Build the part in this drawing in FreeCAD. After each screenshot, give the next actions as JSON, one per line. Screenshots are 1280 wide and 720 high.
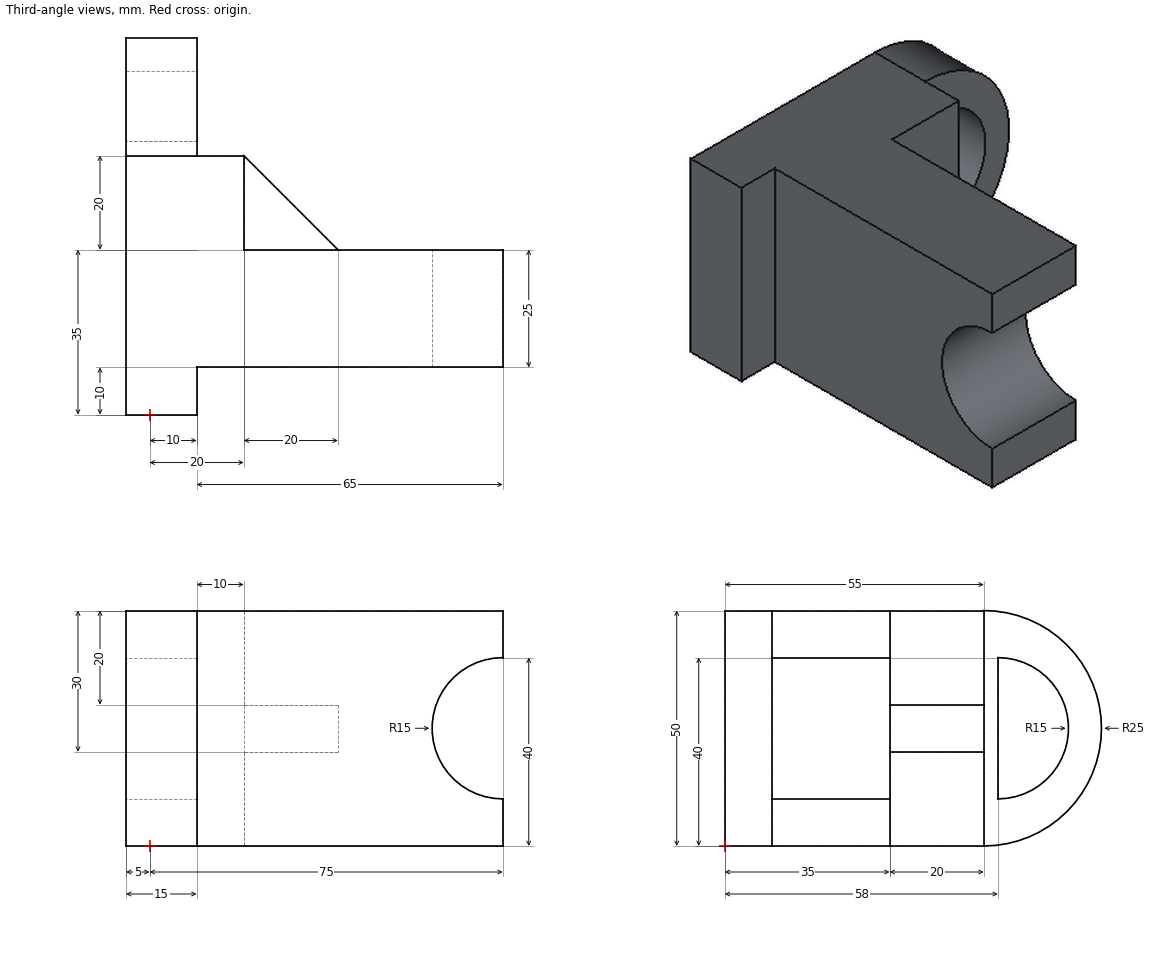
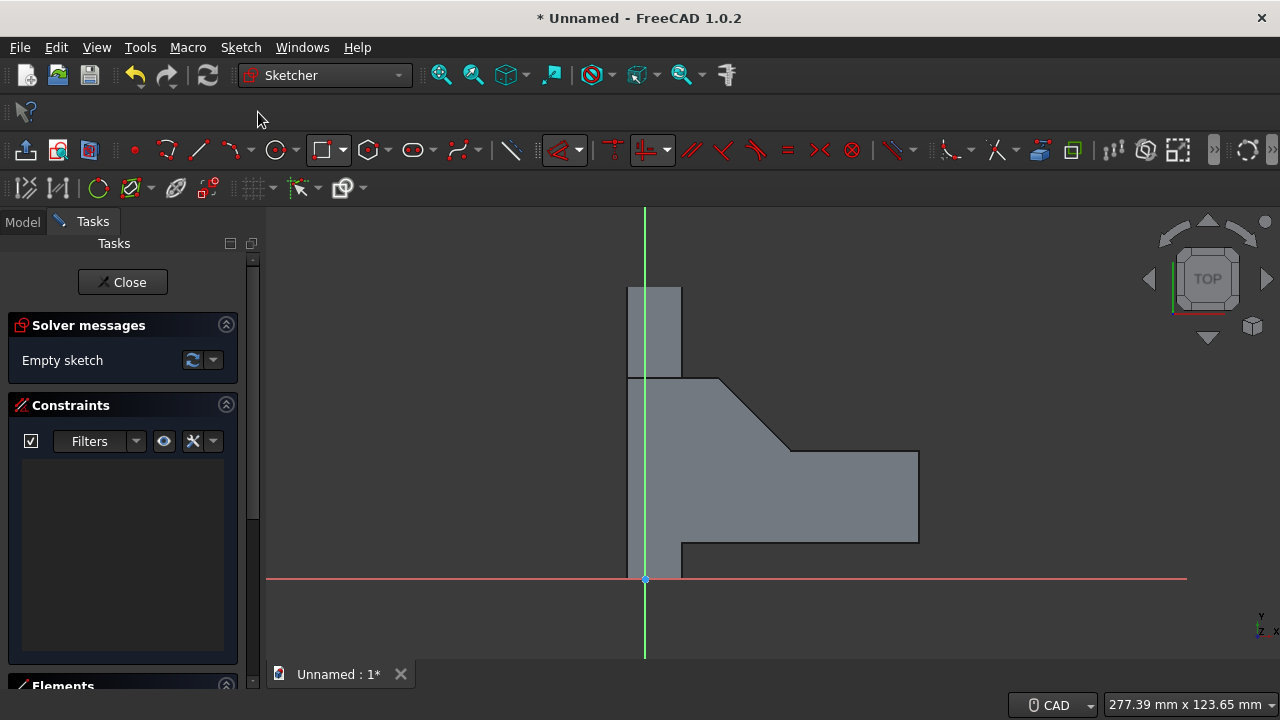
{"action": "scroll", "coordinate": [771, 409], "scroll_direction": "up", "scroll_amount": 7}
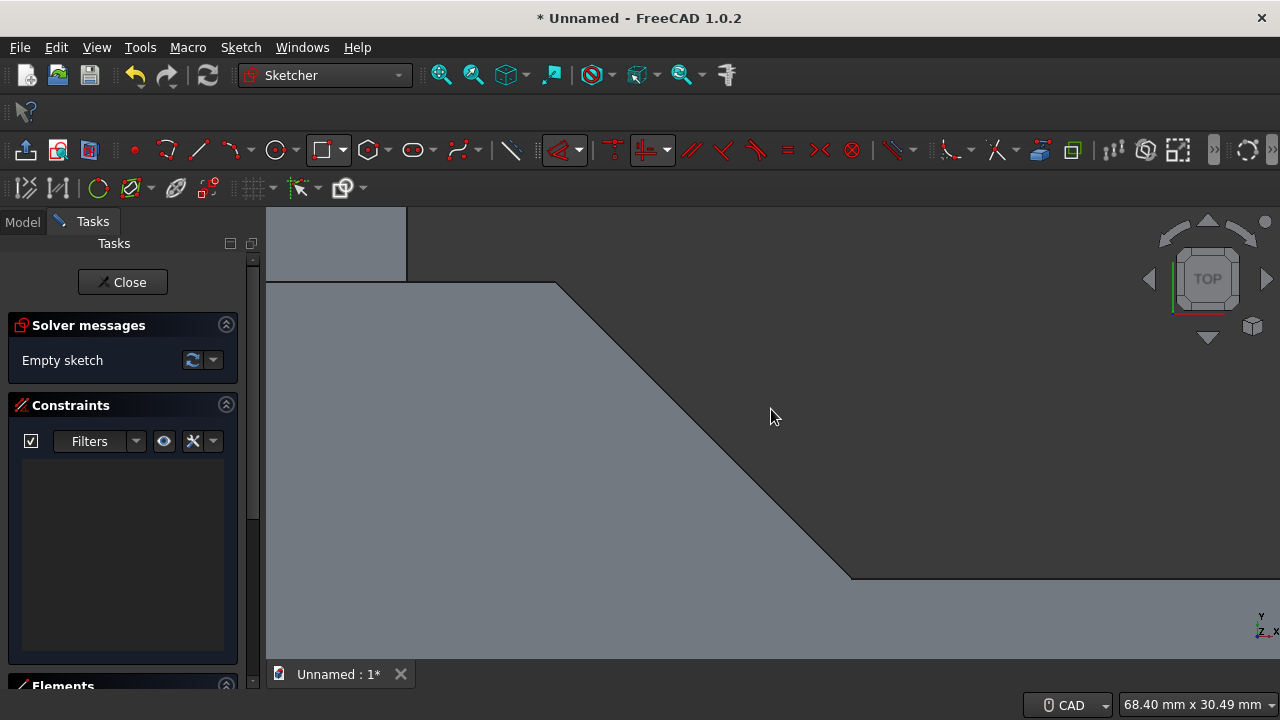
{"action": "left_click", "coordinate": [168, 150]}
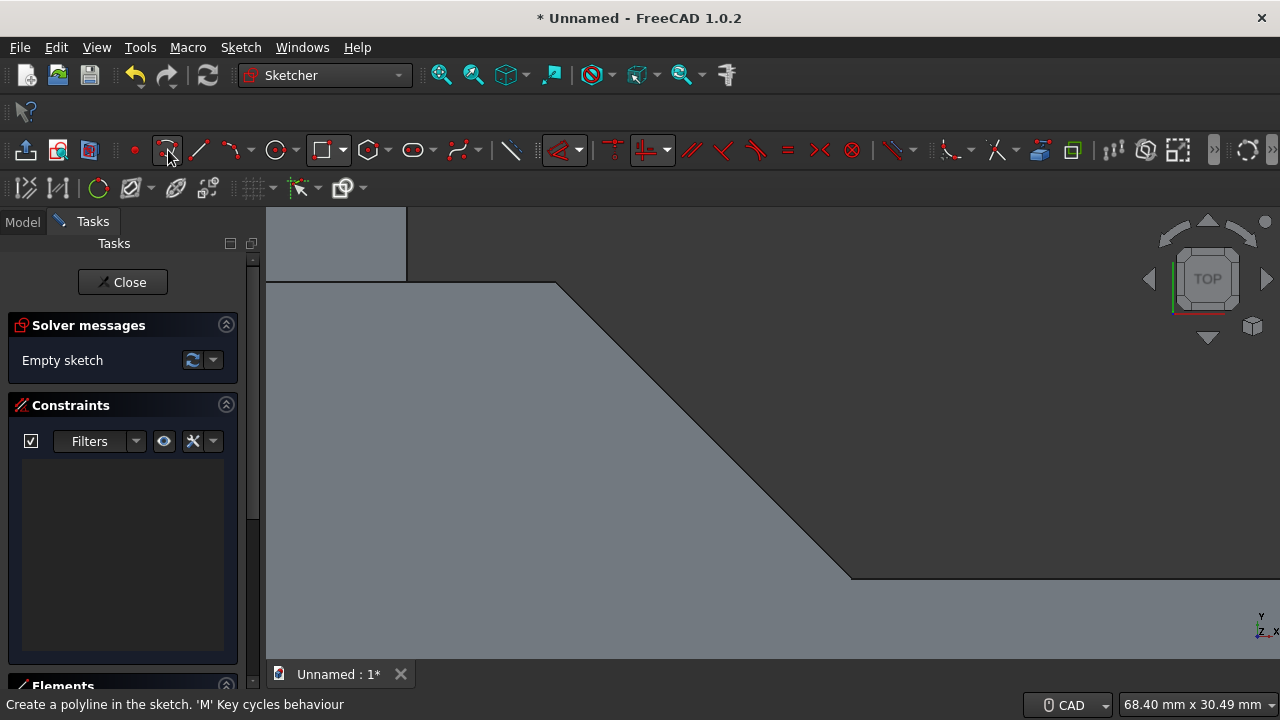
{"action": "left_click", "coordinate": [555, 579]}
{"action": "left_click", "coordinate": [852, 579]}
{"action": "left_click", "coordinate": [555, 282]}
{"action": "left_click", "coordinate": [555, 580]}
{"action": "key", "text": "Escape"}
{"action": "key", "text": "Escape"}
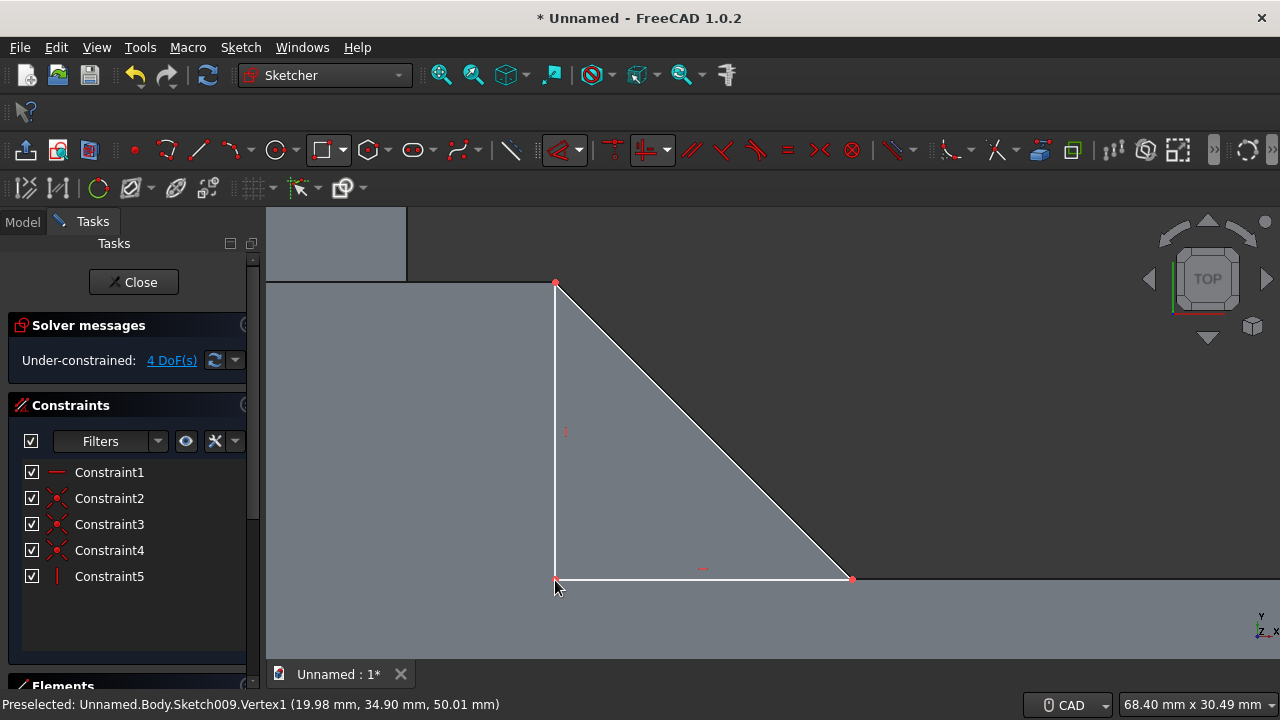
{"action": "left_click", "coordinate": [644, 580]}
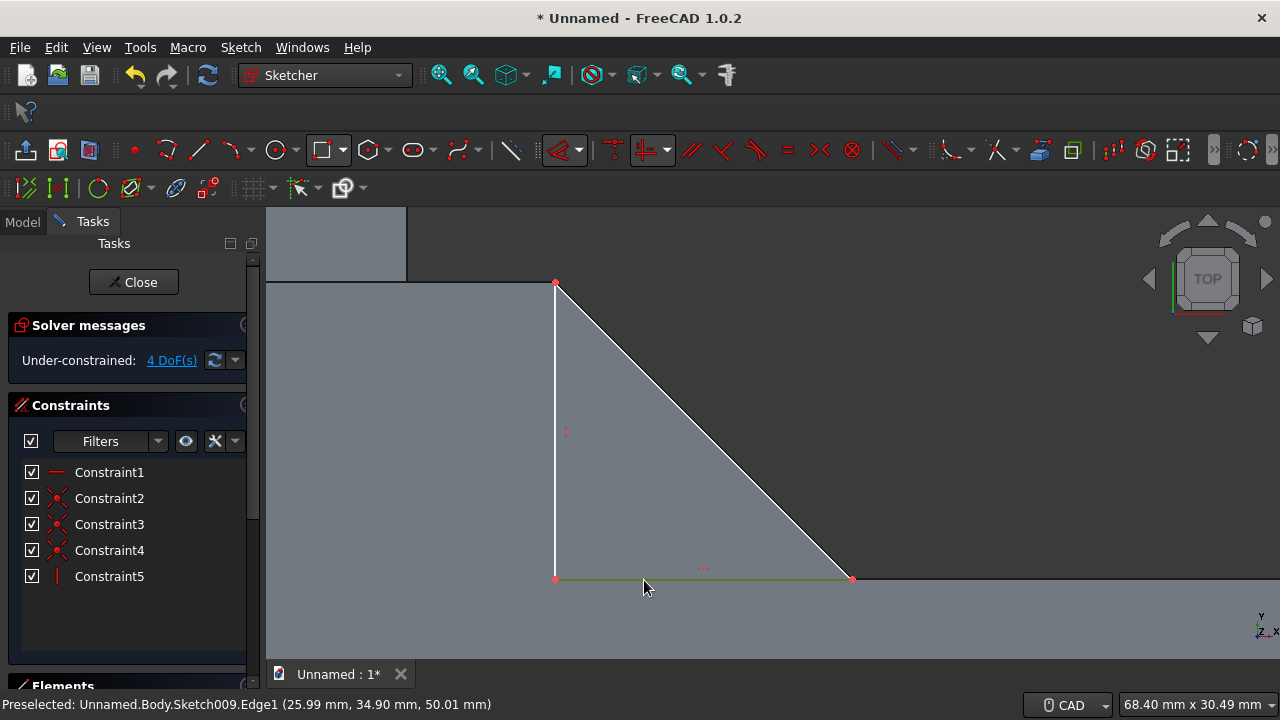
{"action": "left_click", "coordinate": [582, 150]}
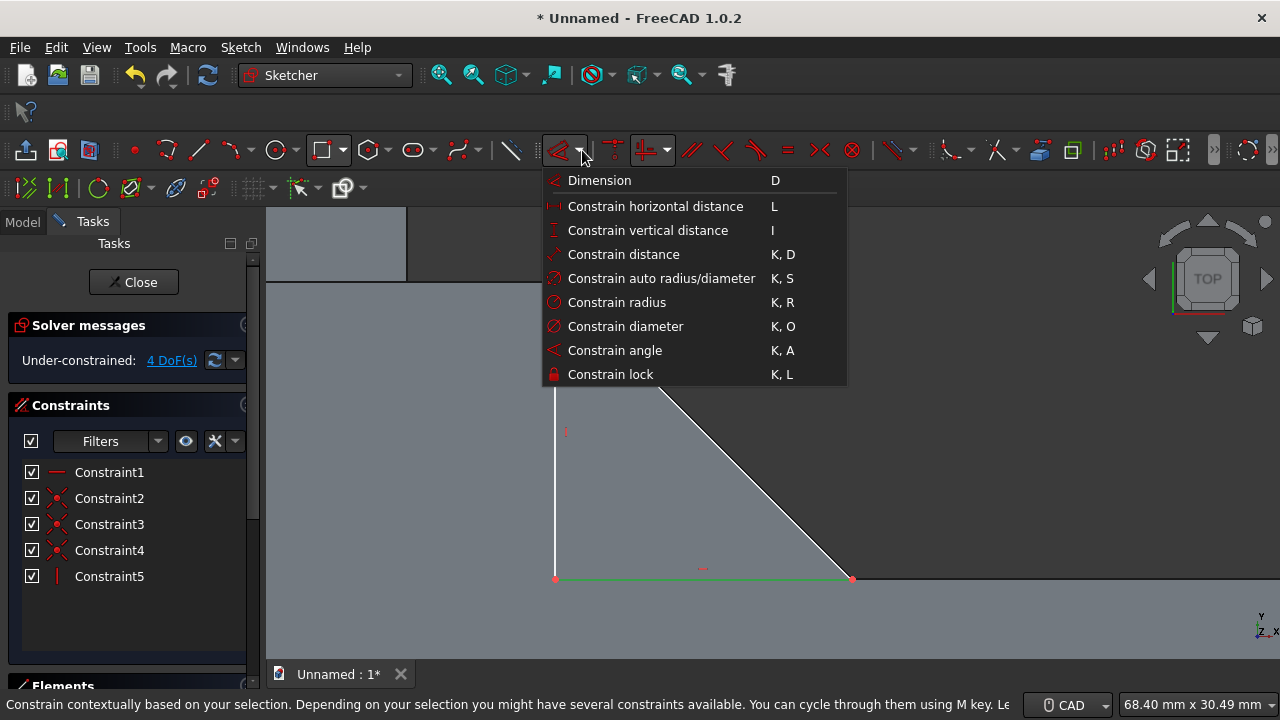
{"action": "left_click", "coordinate": [695, 206]}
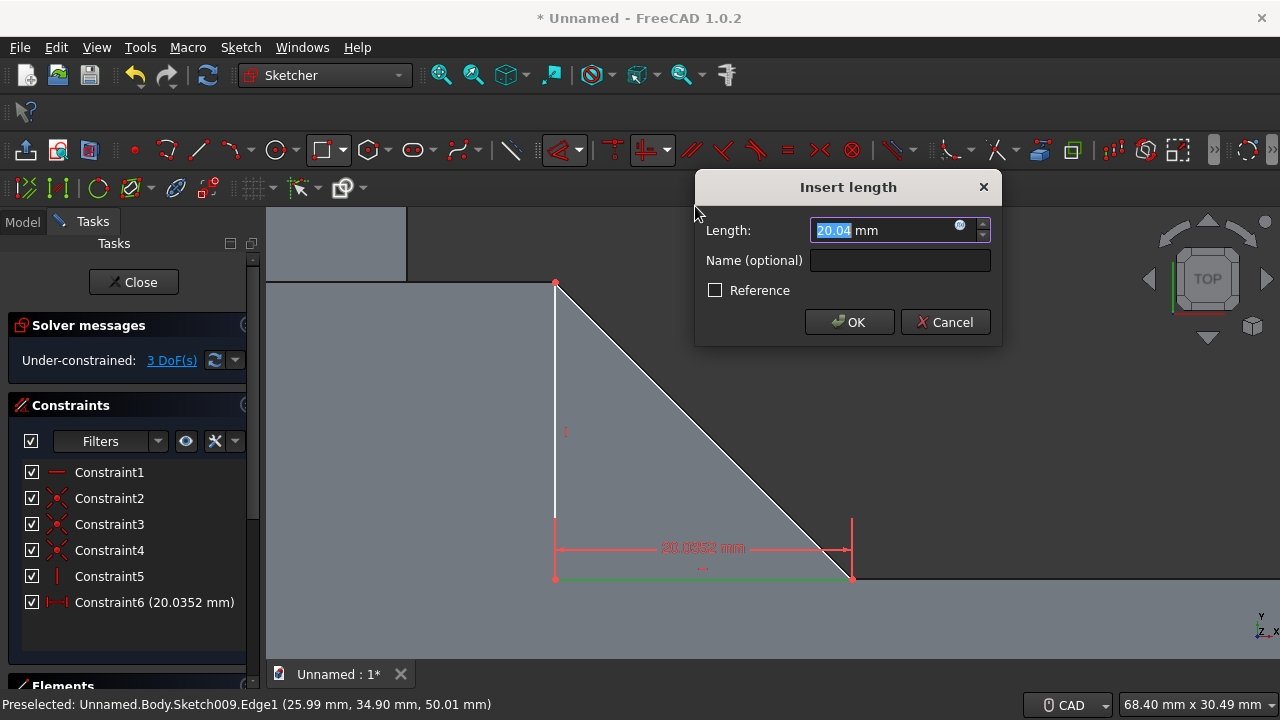
{"action": "type", "text": "20"}
{"action": "key", "text": "Return"}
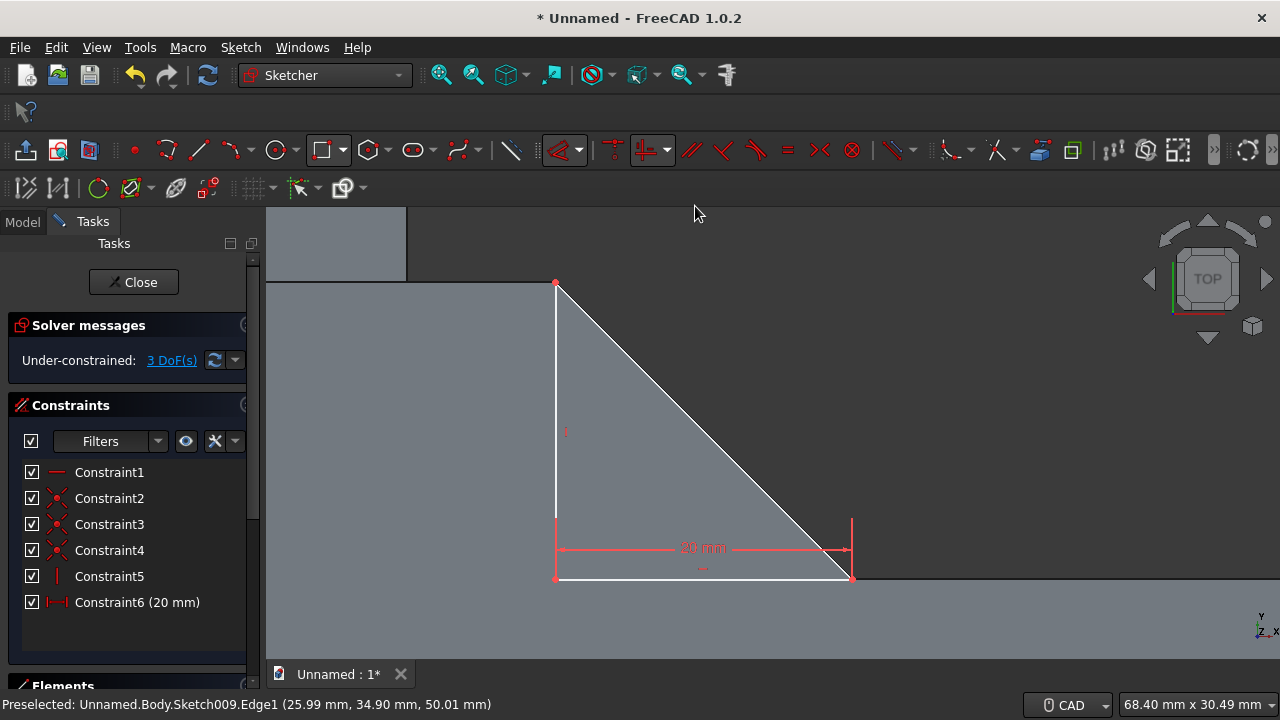
{"action": "left_click", "coordinate": [556, 372]}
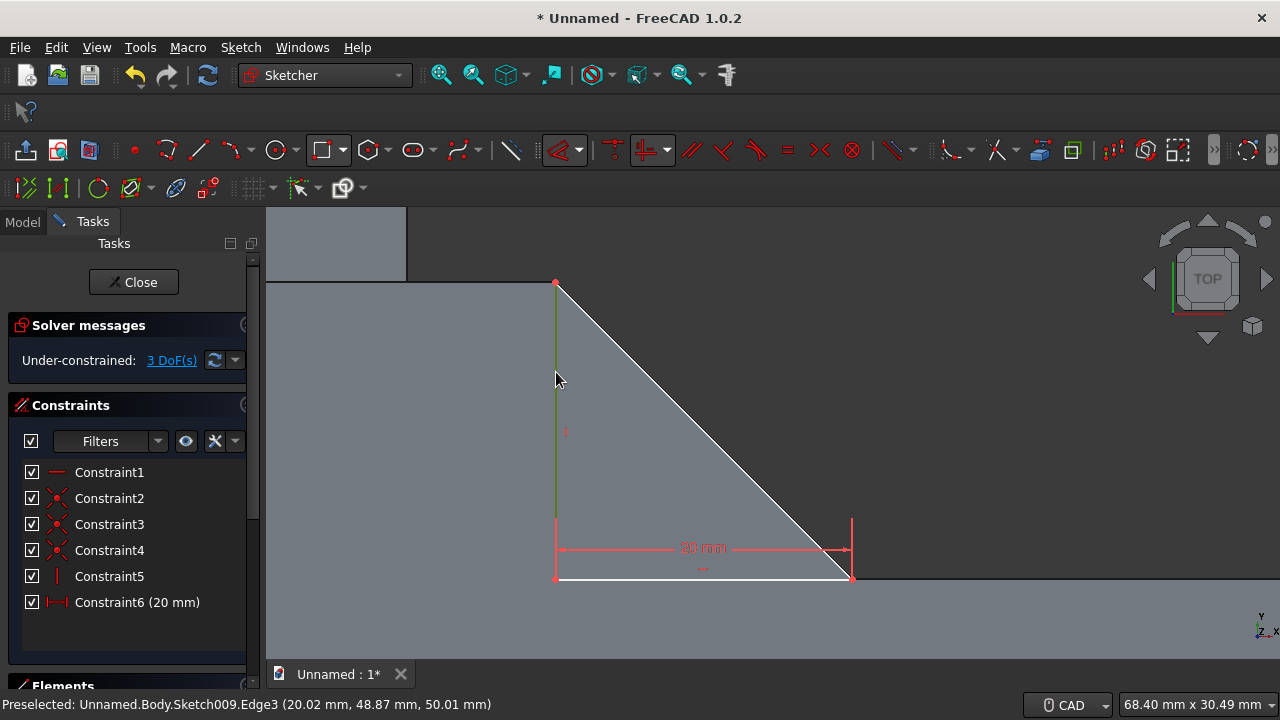
{"action": "key", "text": "i"}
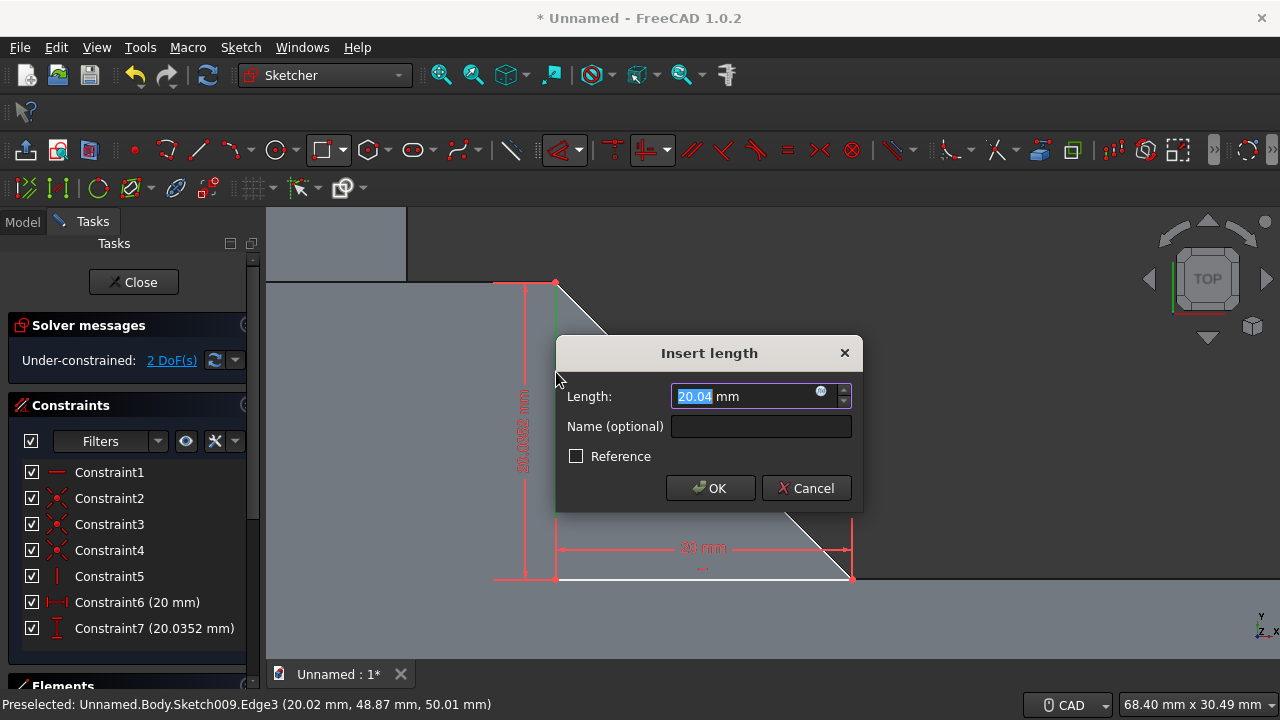
{"action": "type", "text": "20"}
{"action": "key", "text": "Return"}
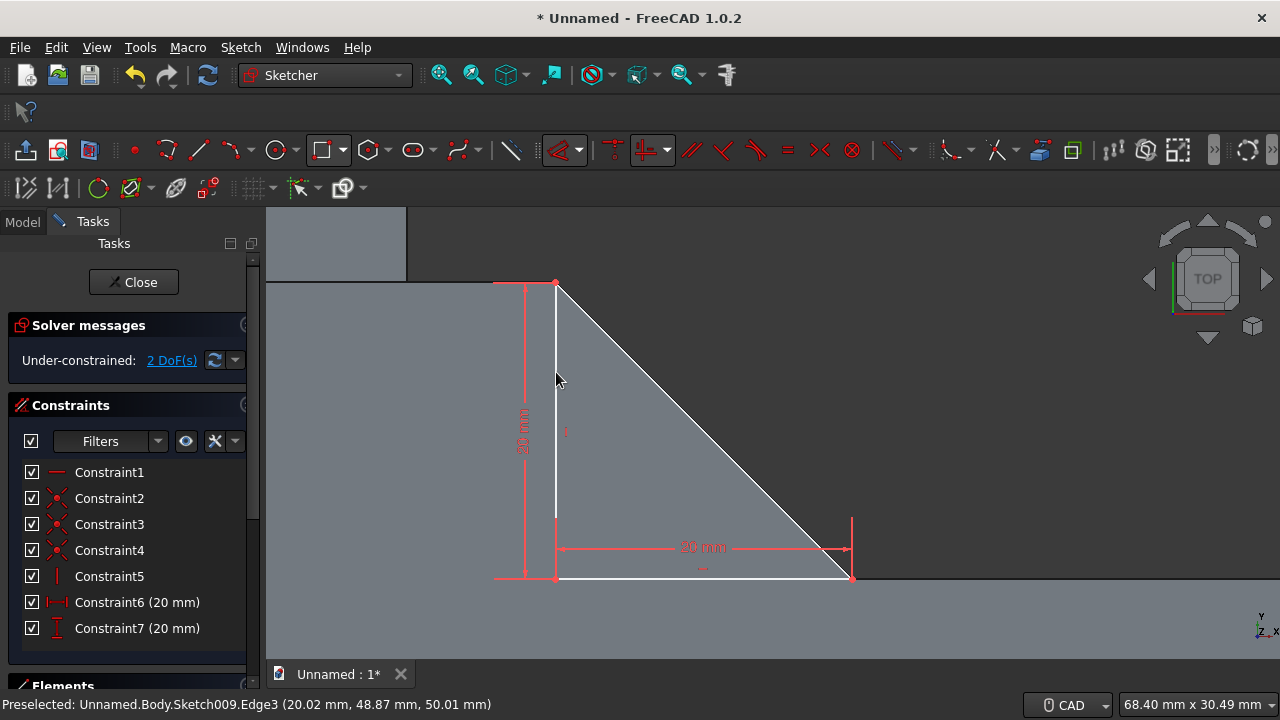
{"action": "left_click", "coordinate": [556, 579]}